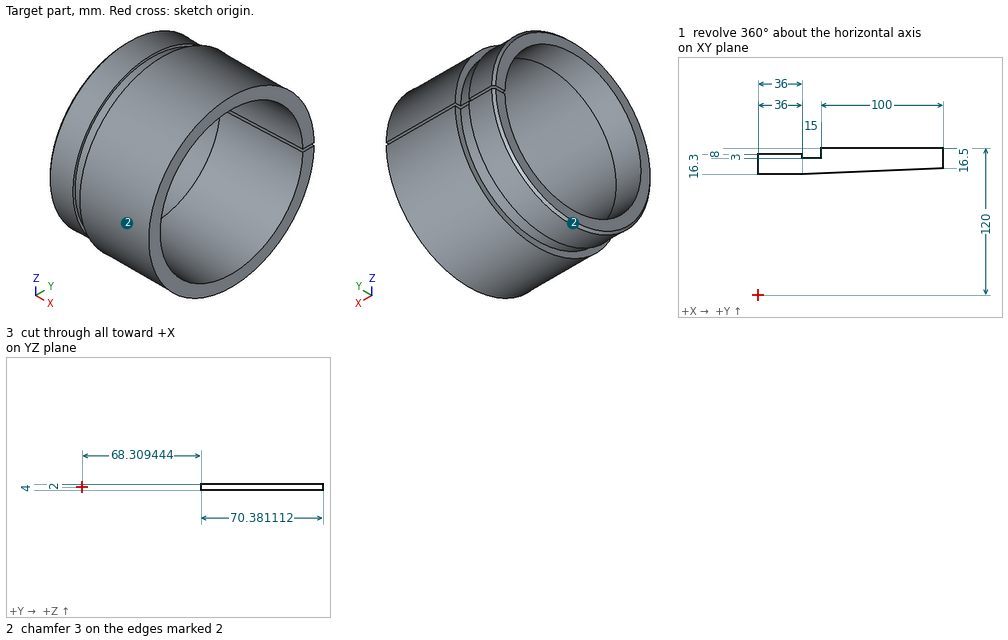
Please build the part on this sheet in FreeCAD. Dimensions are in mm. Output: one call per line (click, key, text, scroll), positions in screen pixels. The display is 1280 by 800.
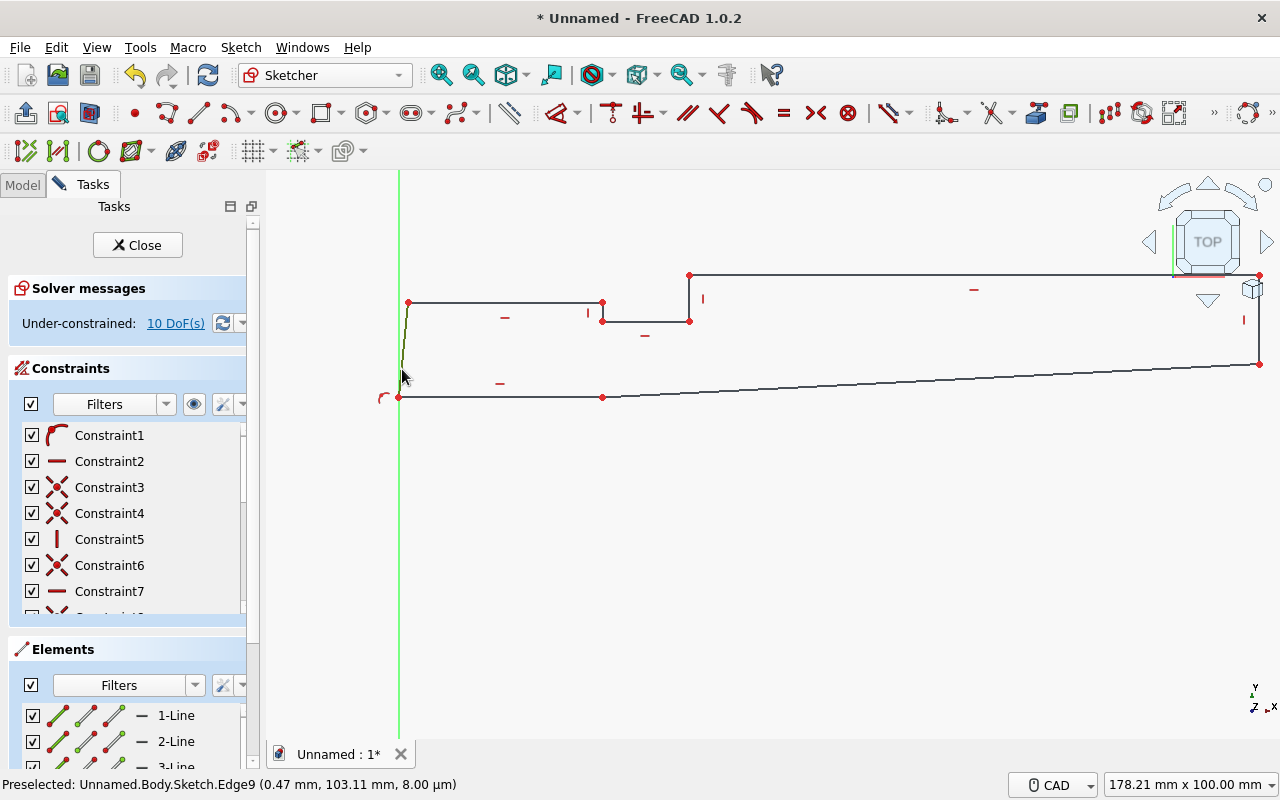
click(666, 114)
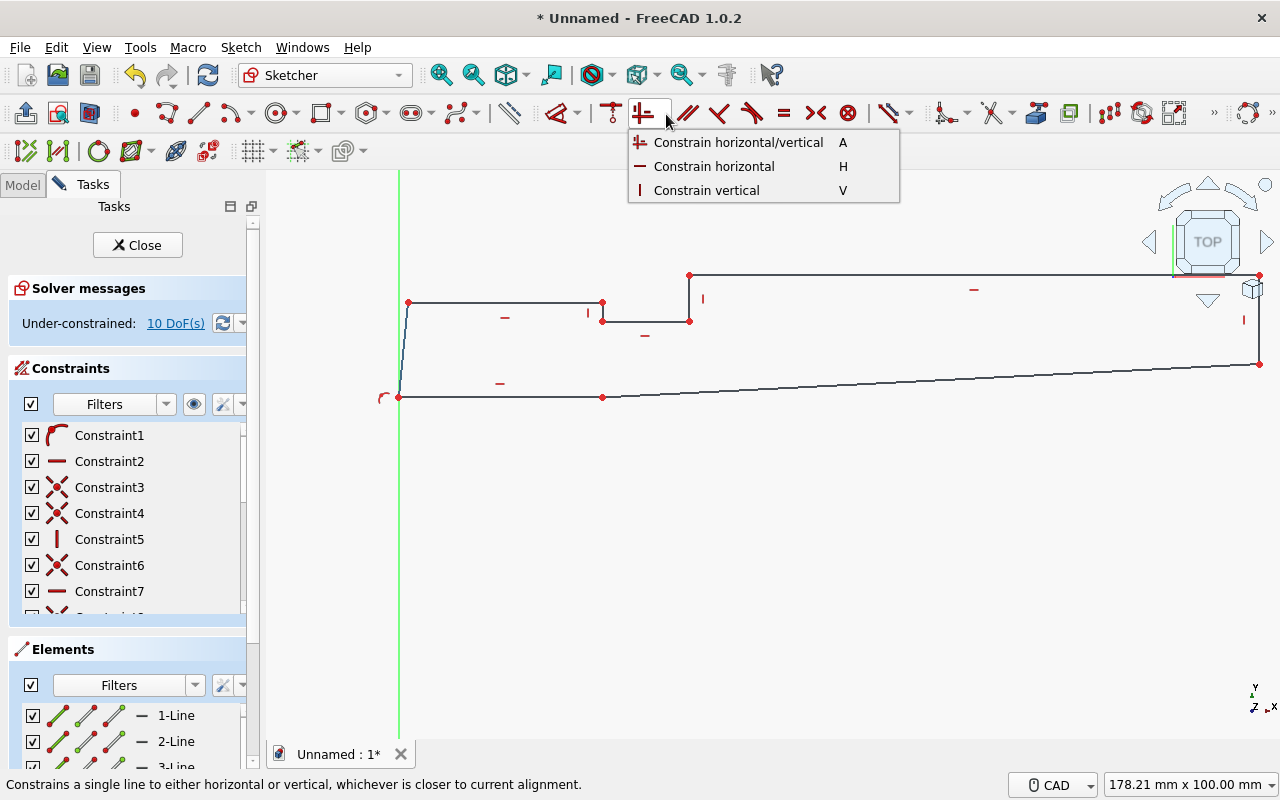
click(764, 190)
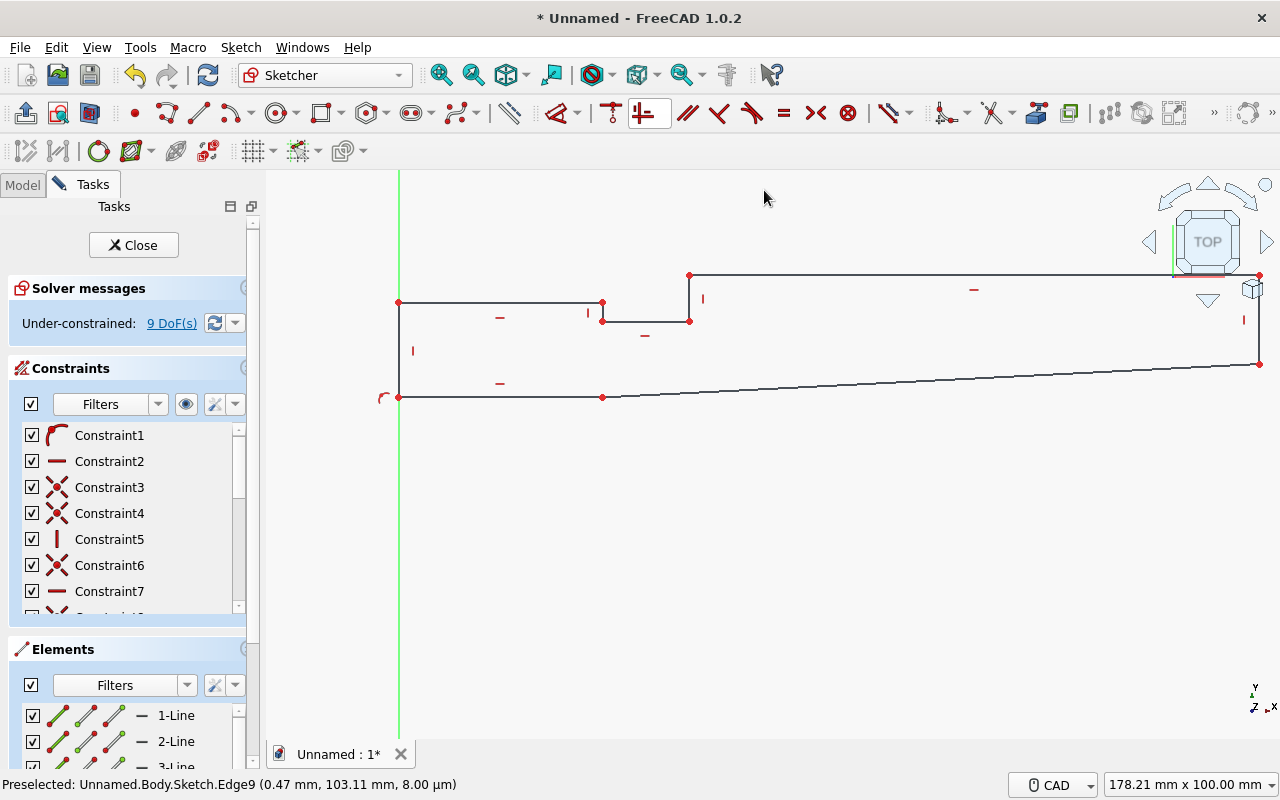
click(689, 289)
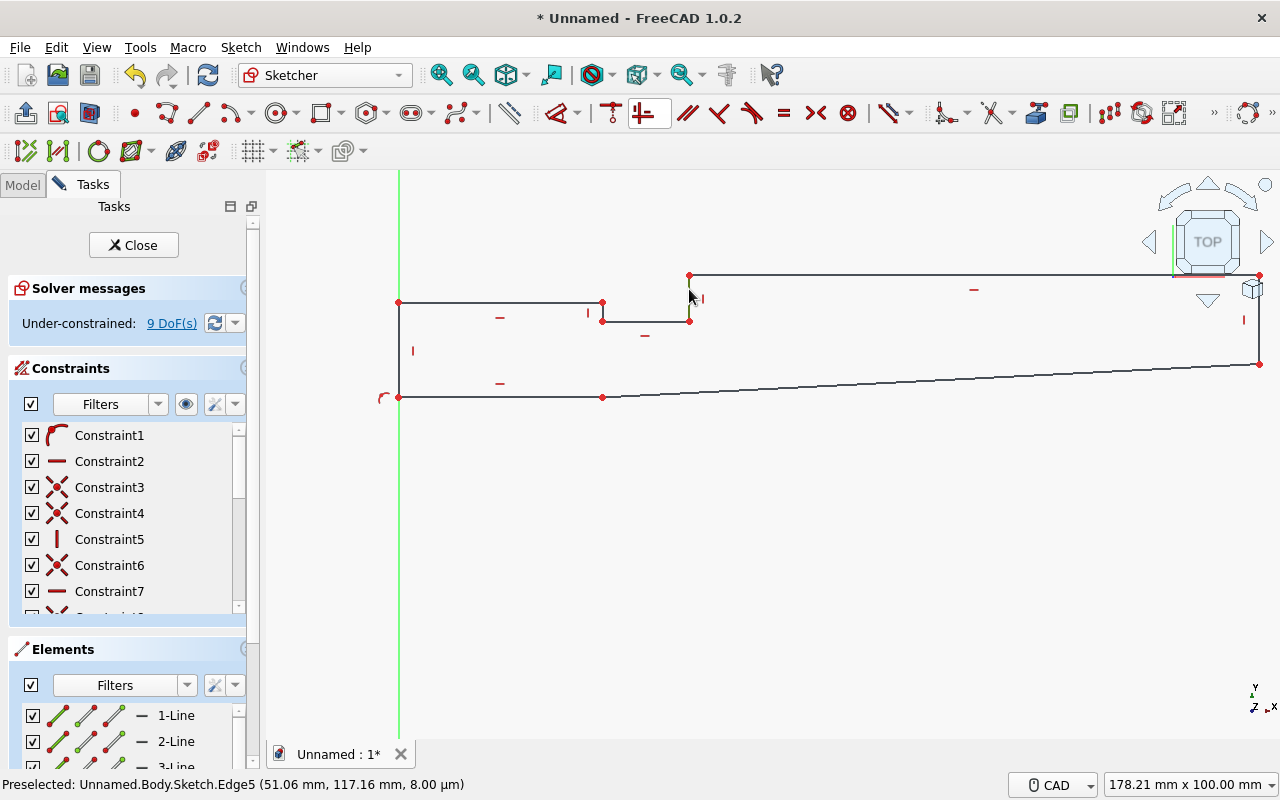
key(i)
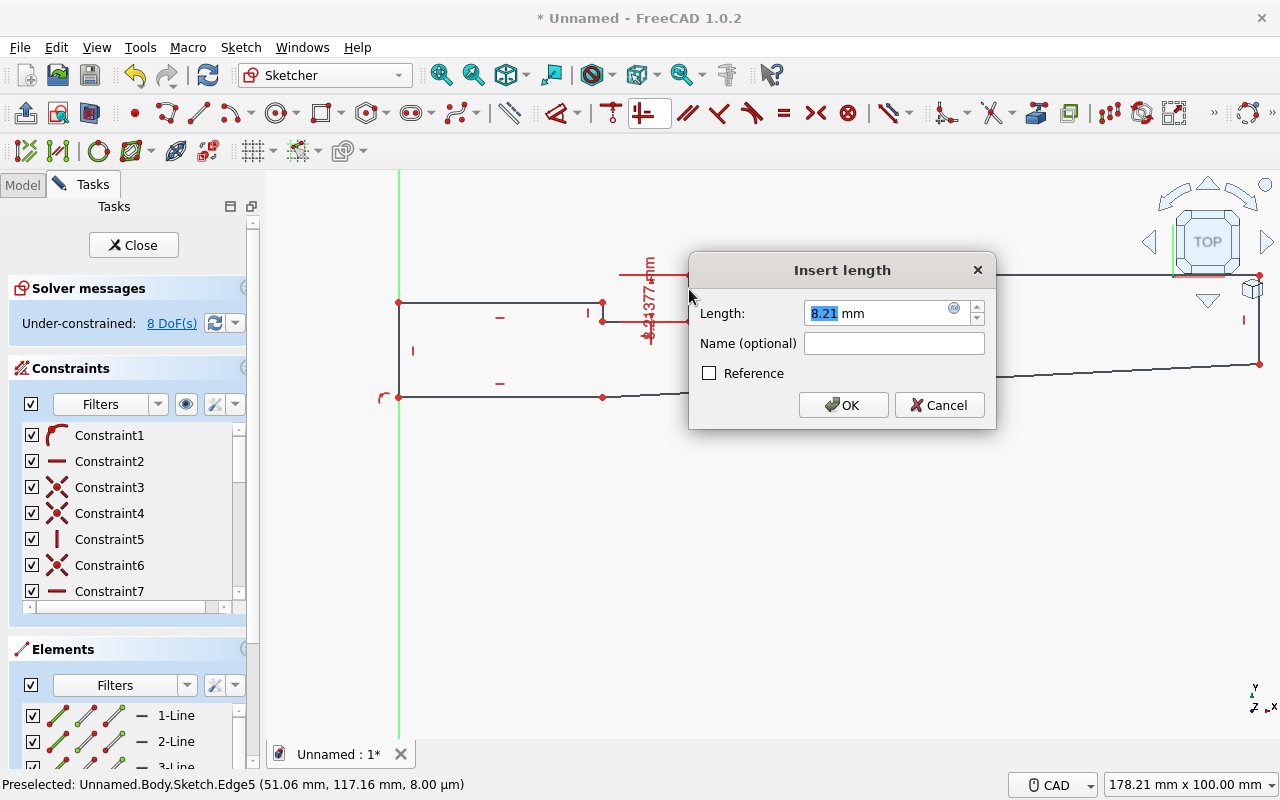
text(8)
key(Return)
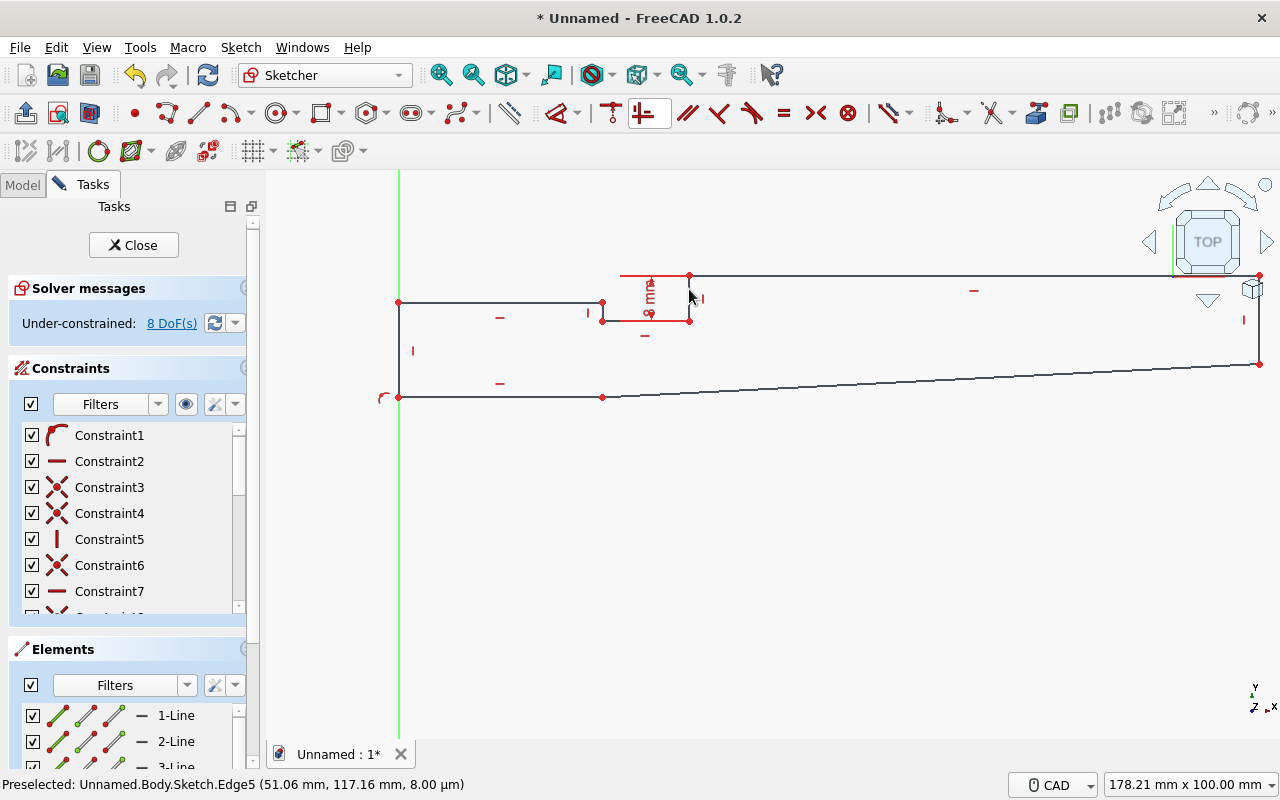
scroll(603, 312, up, 5)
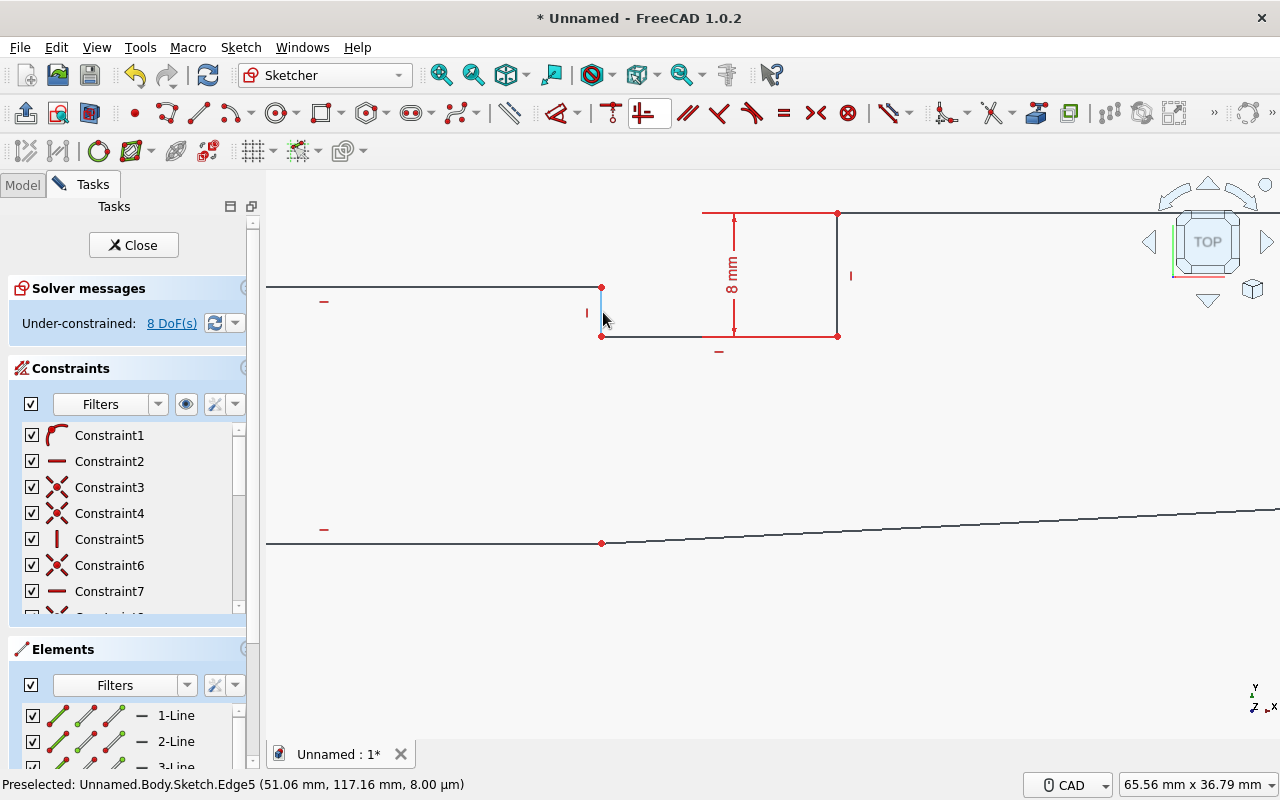
click(601, 312)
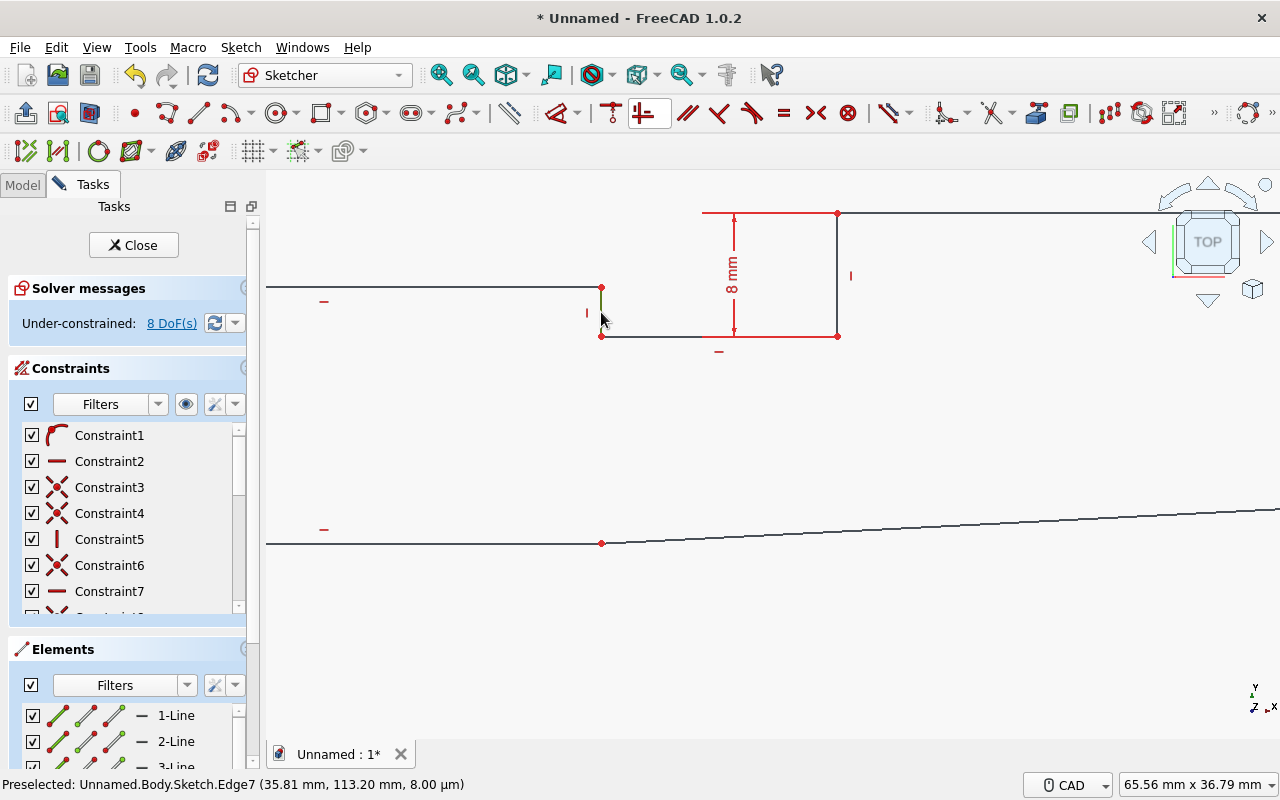
click(580, 114)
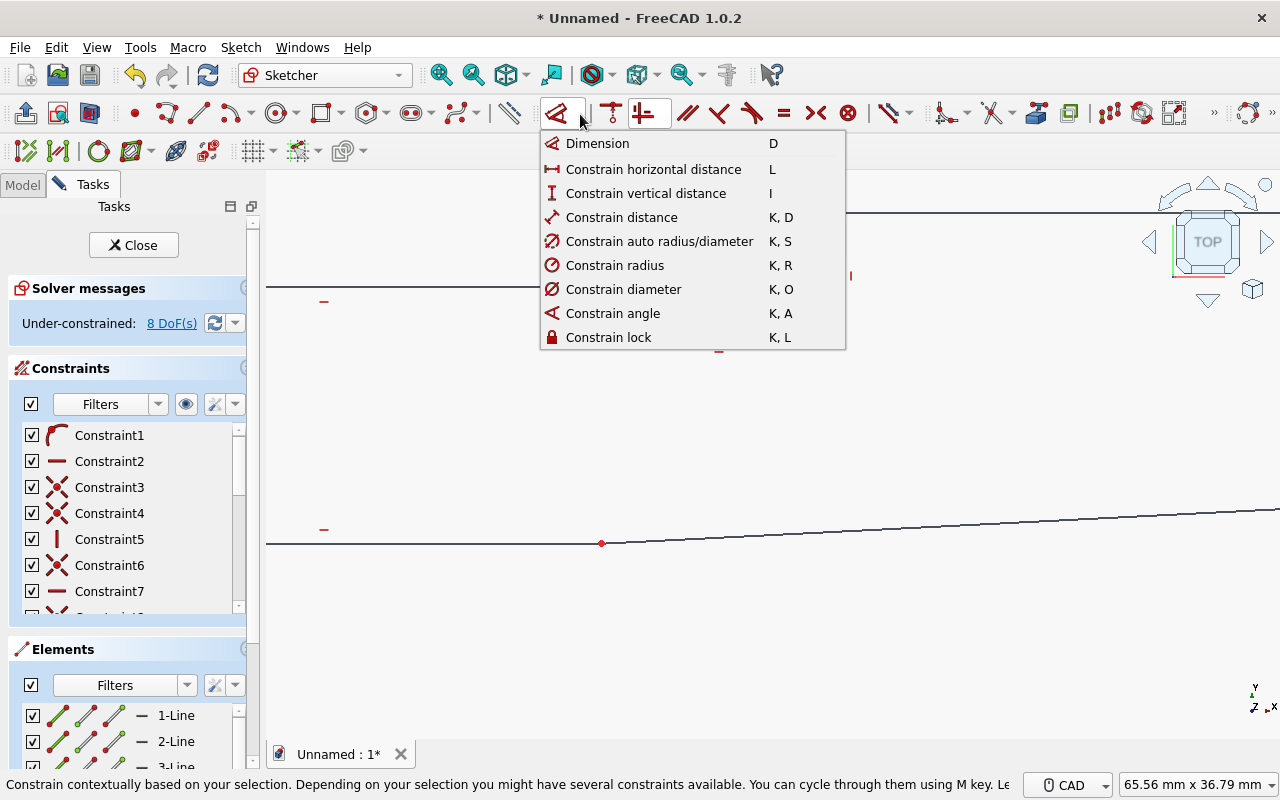
click(693, 193)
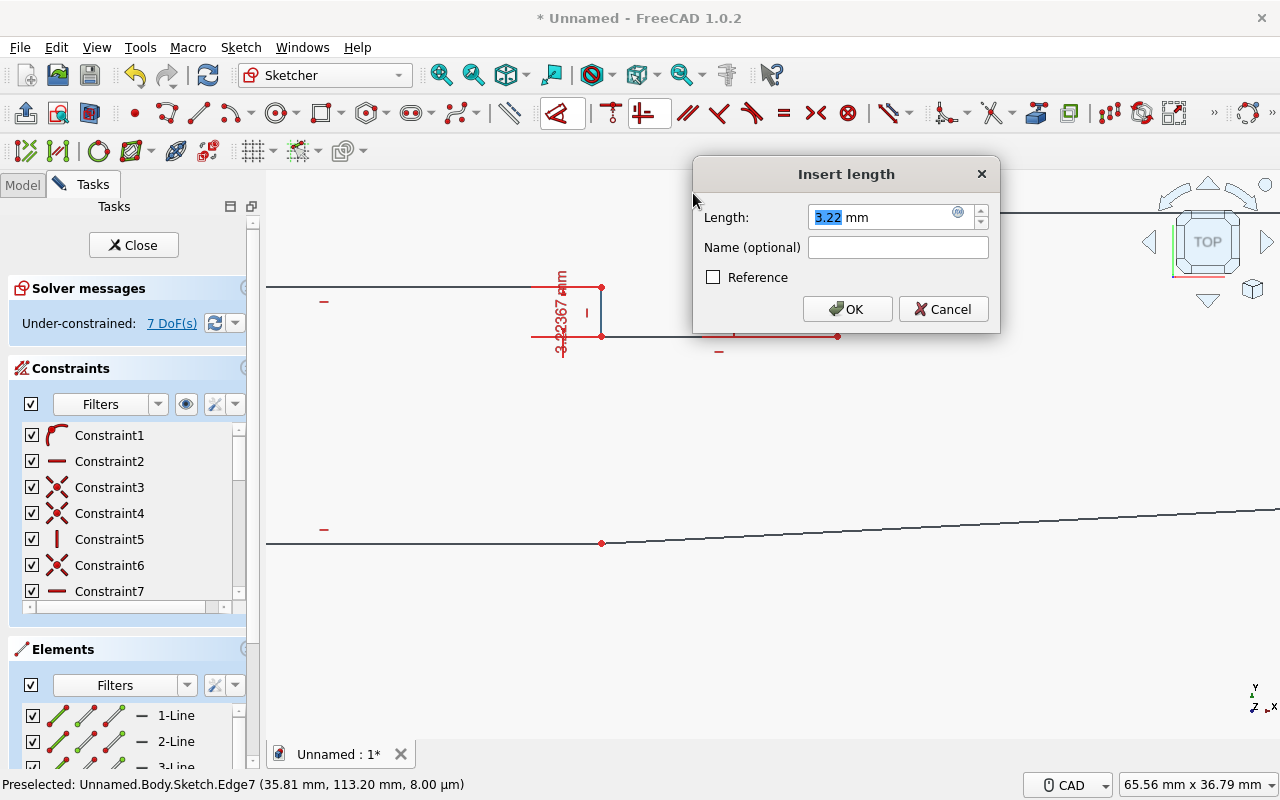
text(3)
key(Return)